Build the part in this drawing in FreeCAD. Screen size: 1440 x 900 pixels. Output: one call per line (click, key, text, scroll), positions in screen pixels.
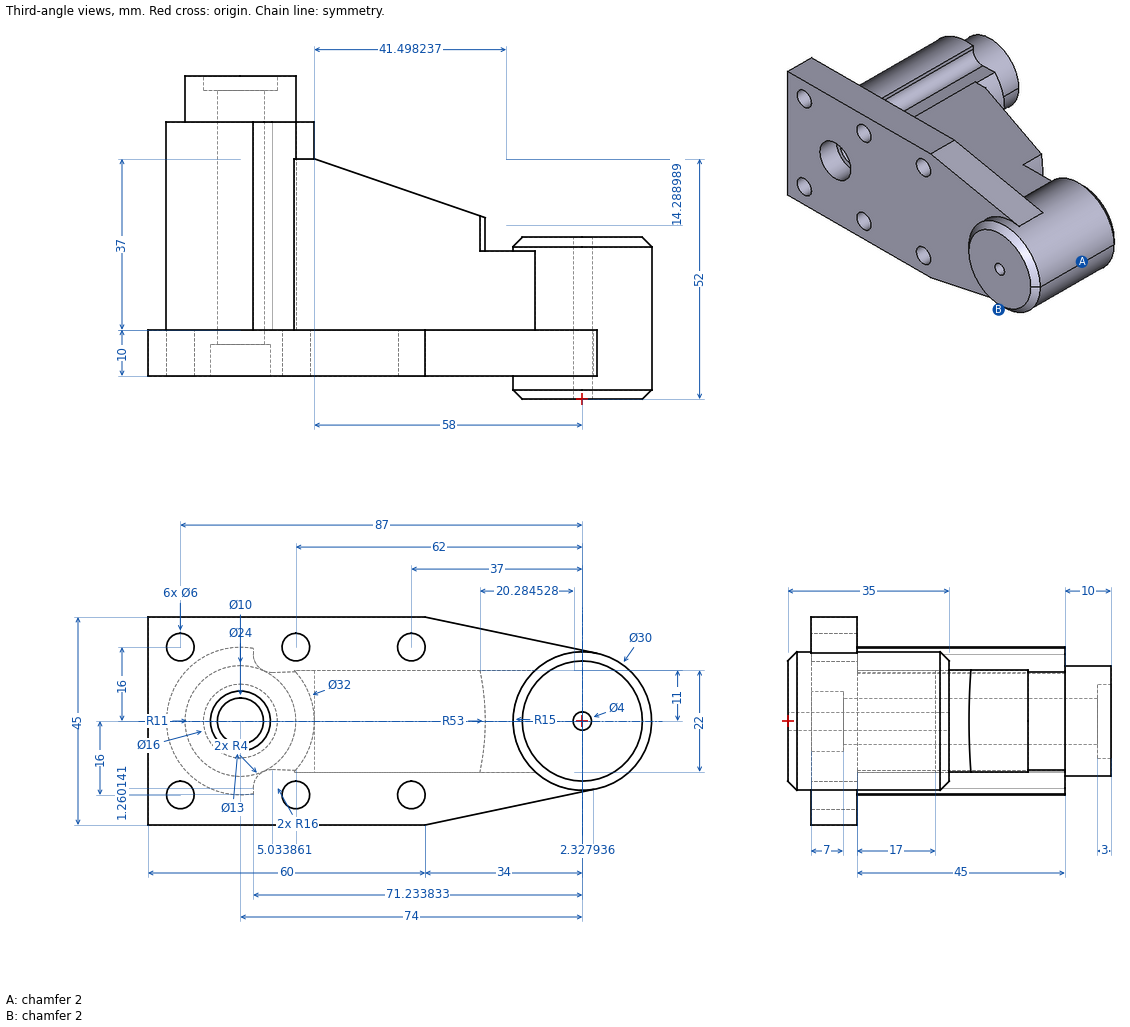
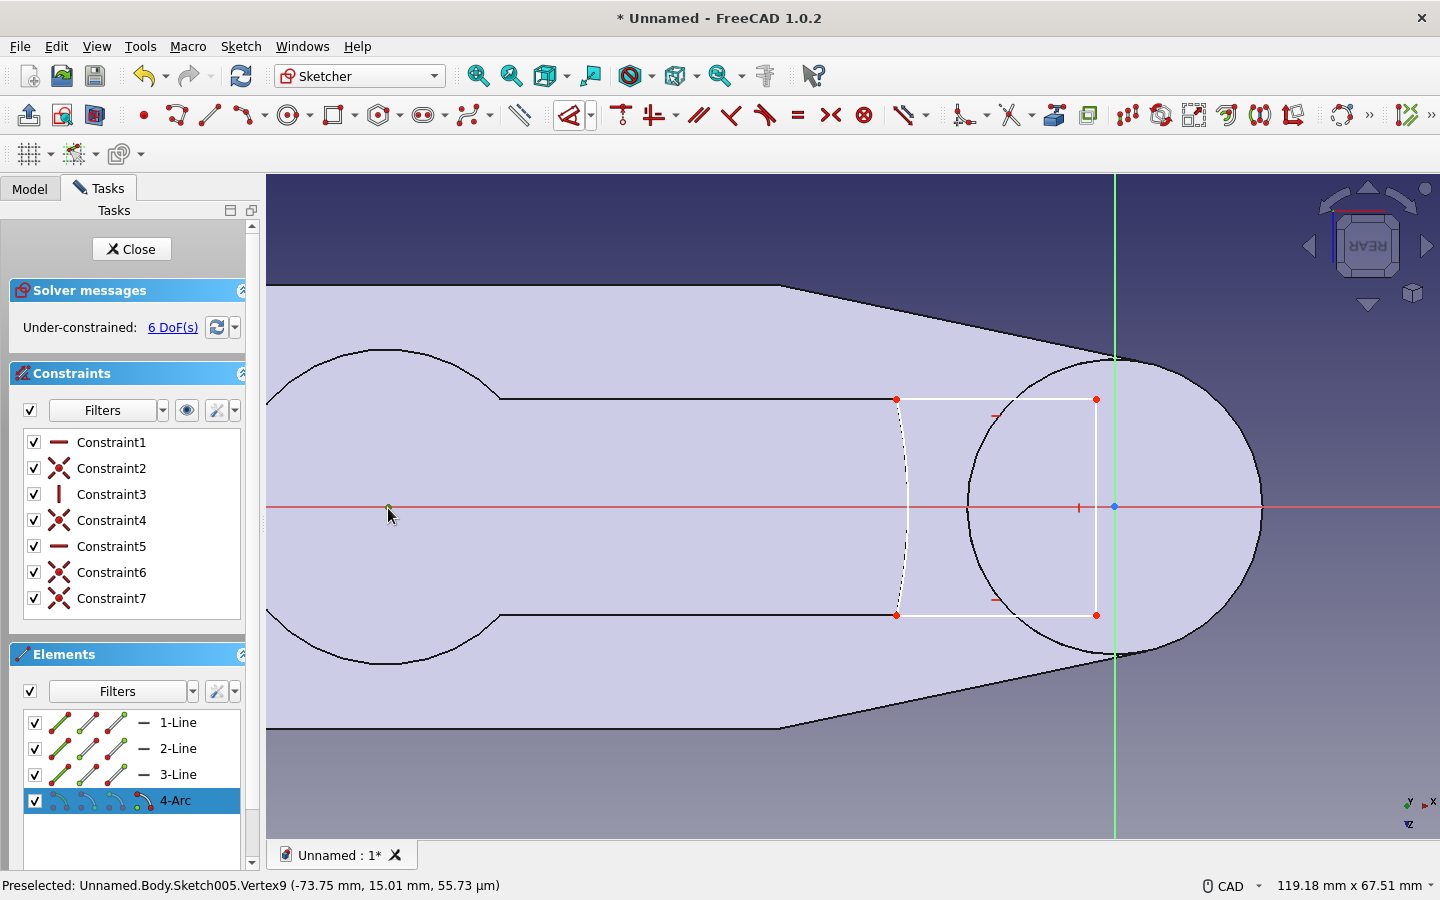
click(364, 507)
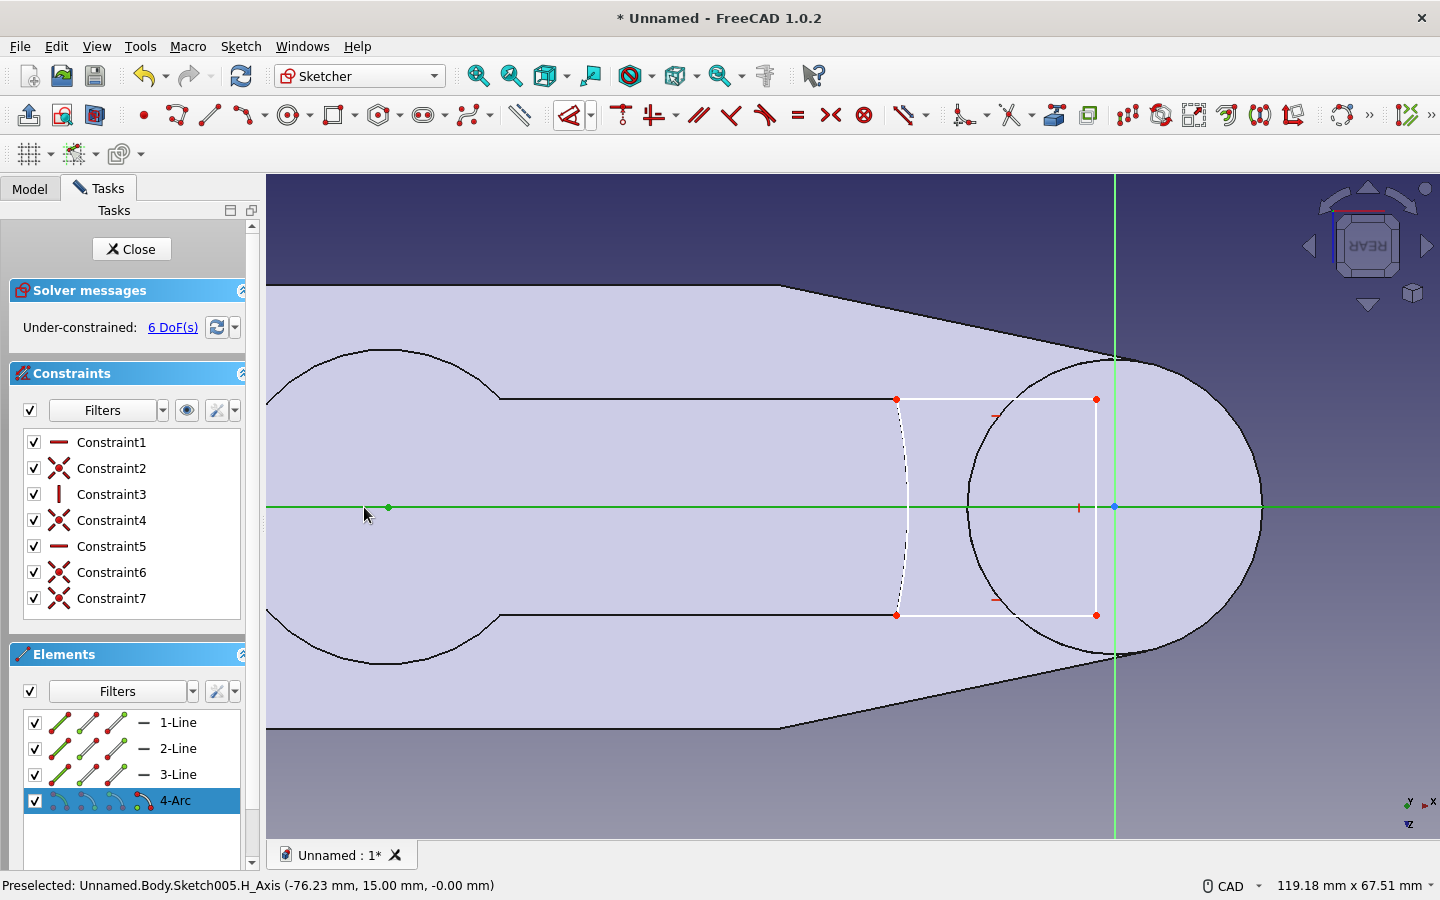
click(621, 116)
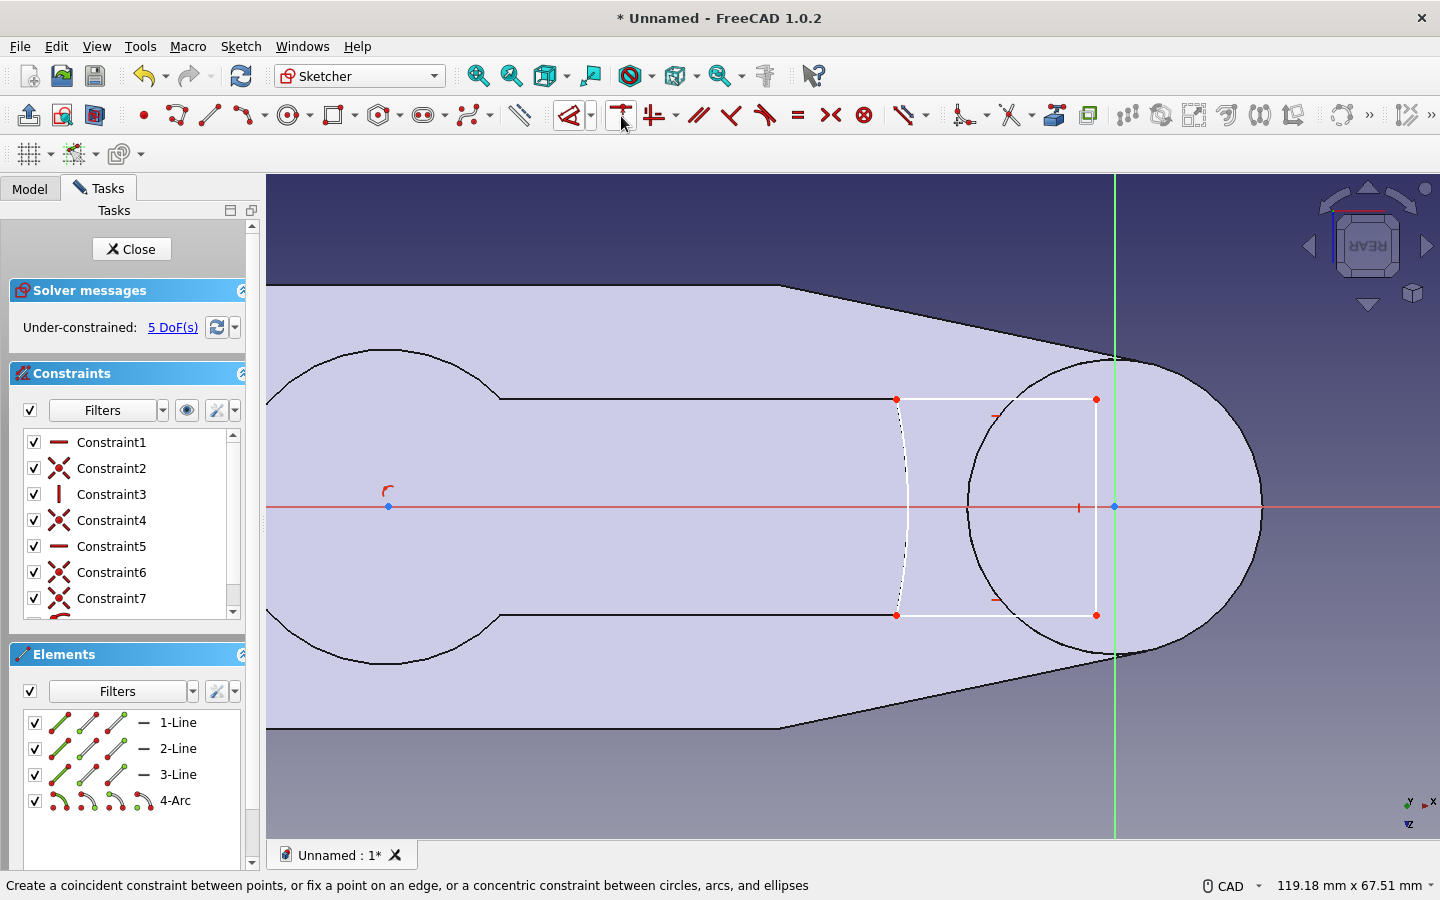
click(906, 551)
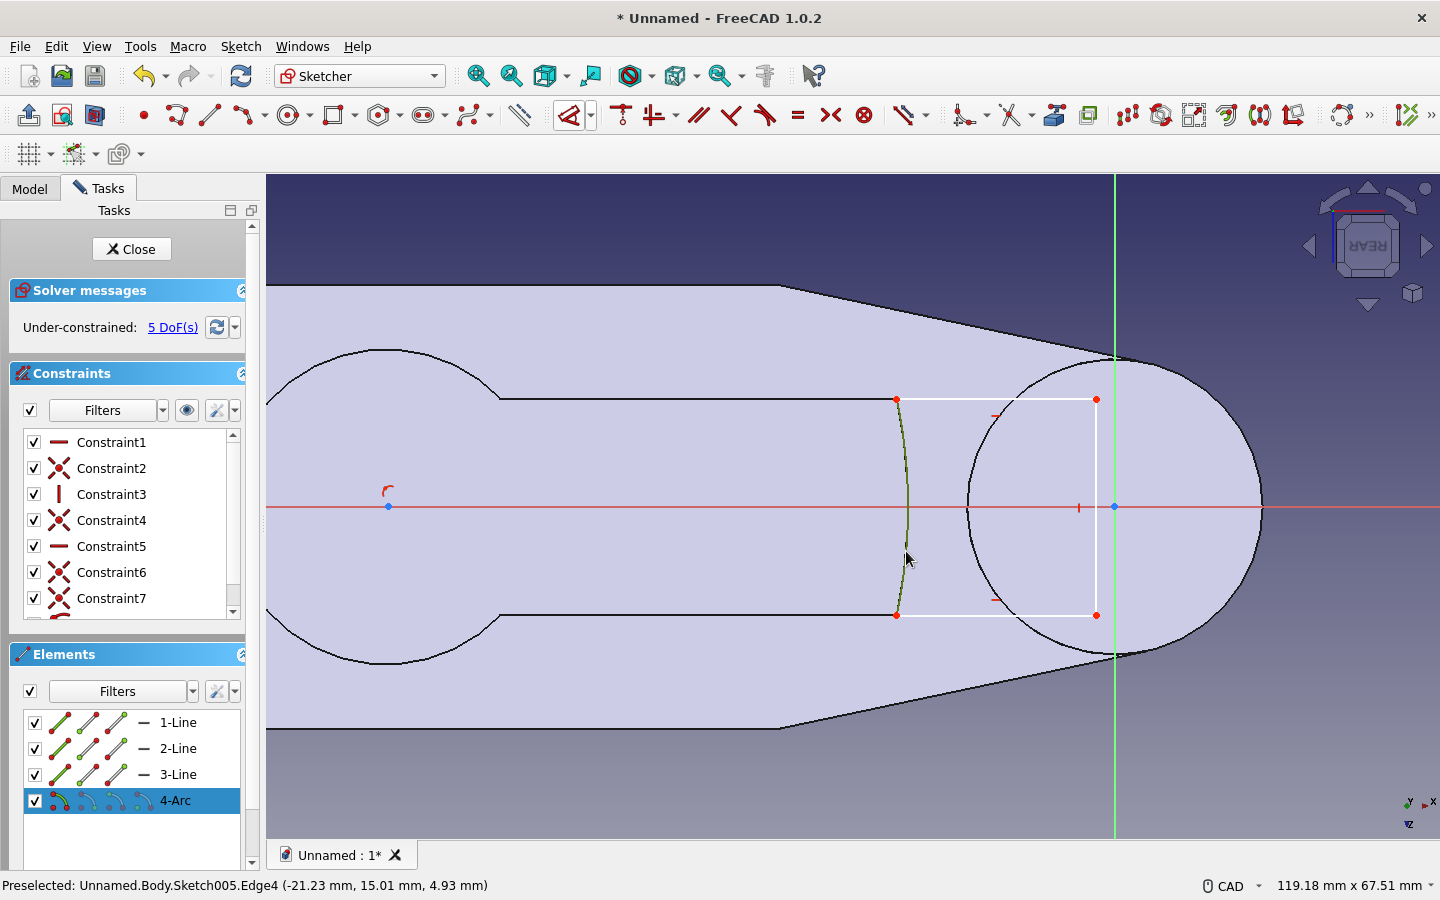
click(590, 116)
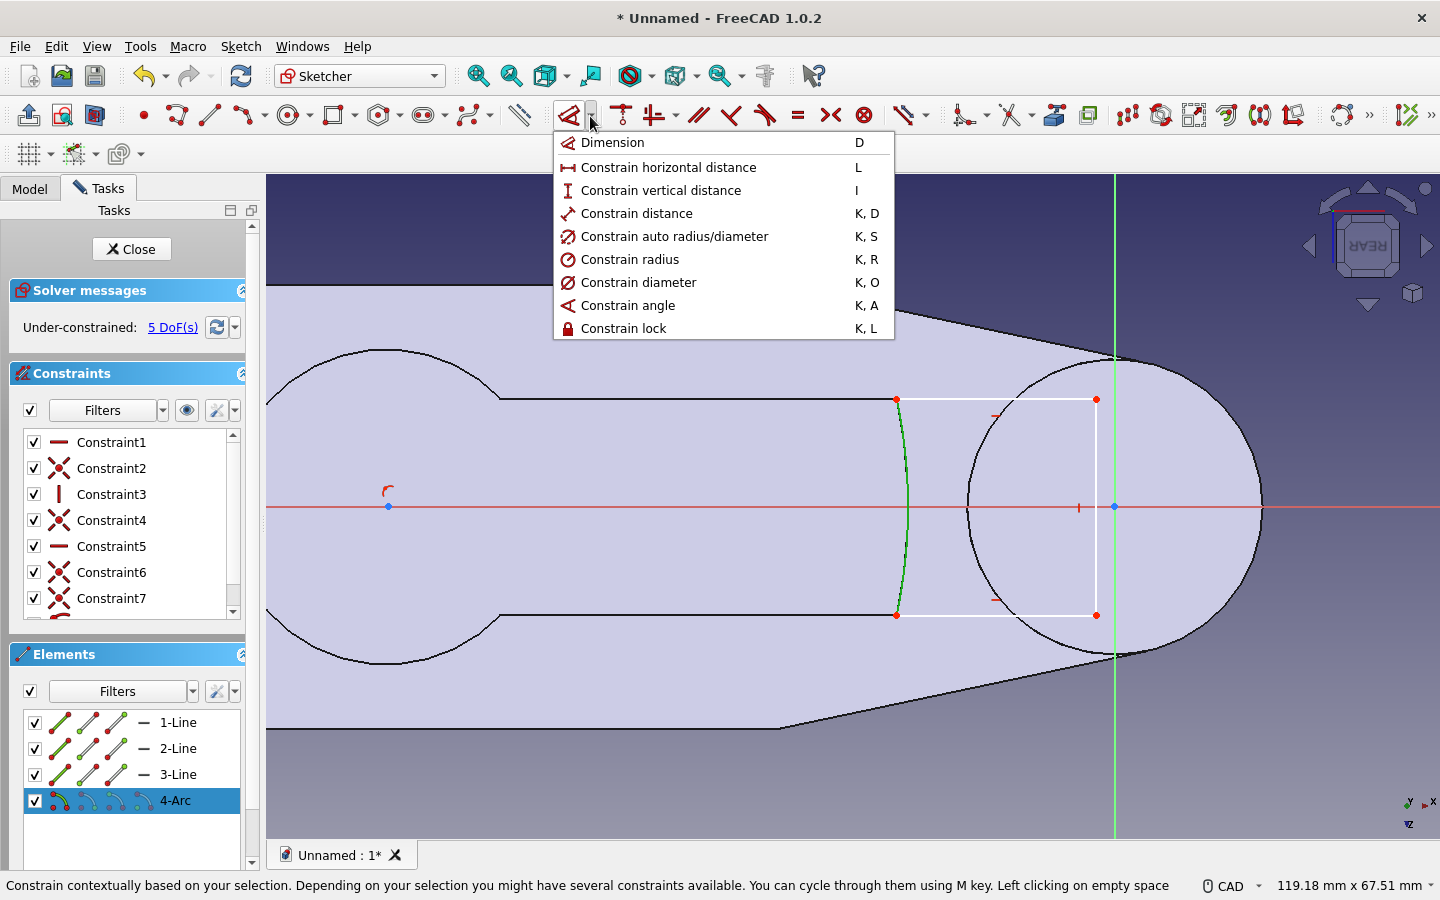
click(724, 260)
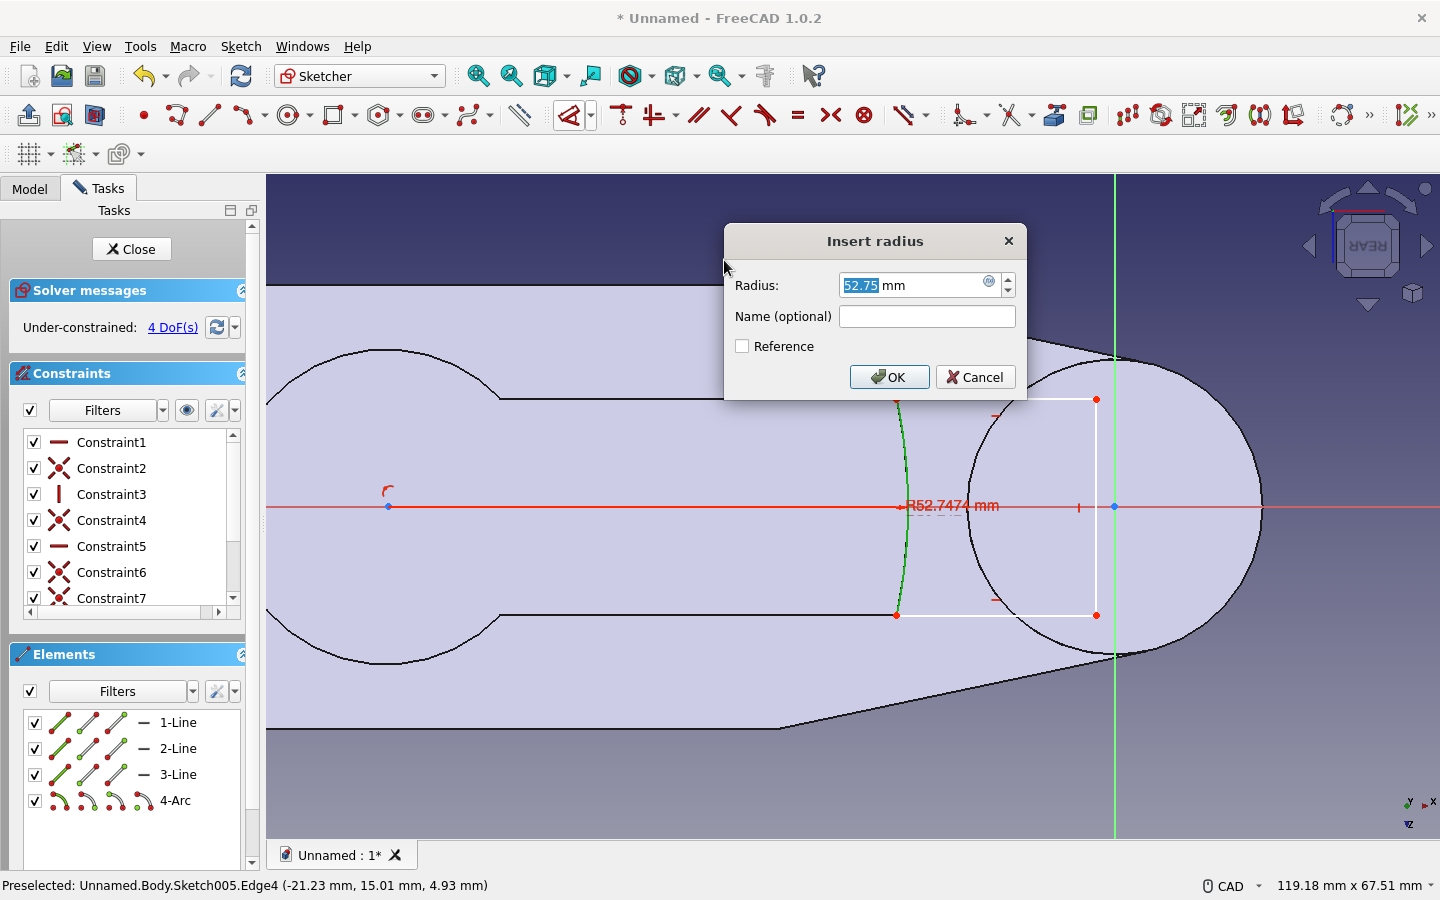
text(53)
key(Return)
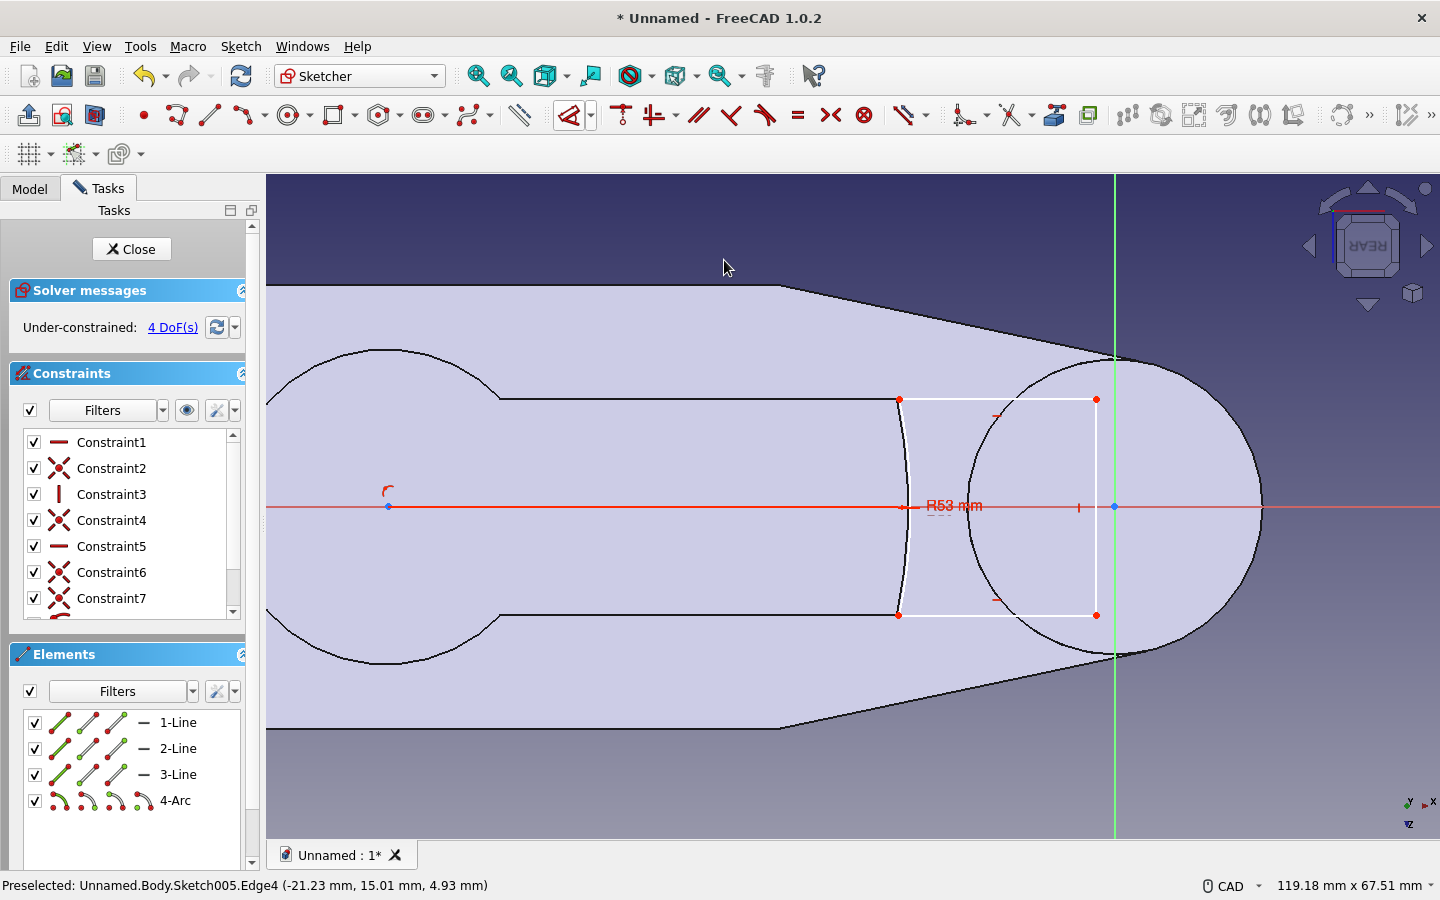
click(1096, 551)